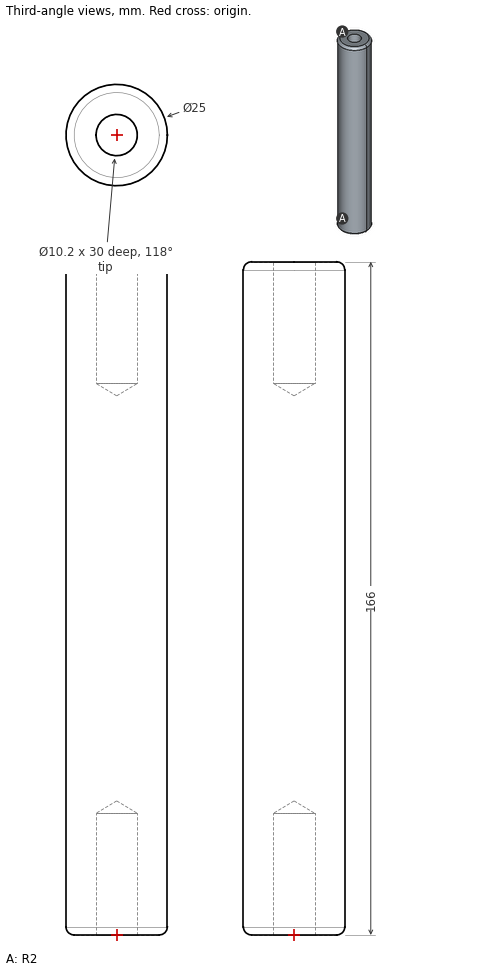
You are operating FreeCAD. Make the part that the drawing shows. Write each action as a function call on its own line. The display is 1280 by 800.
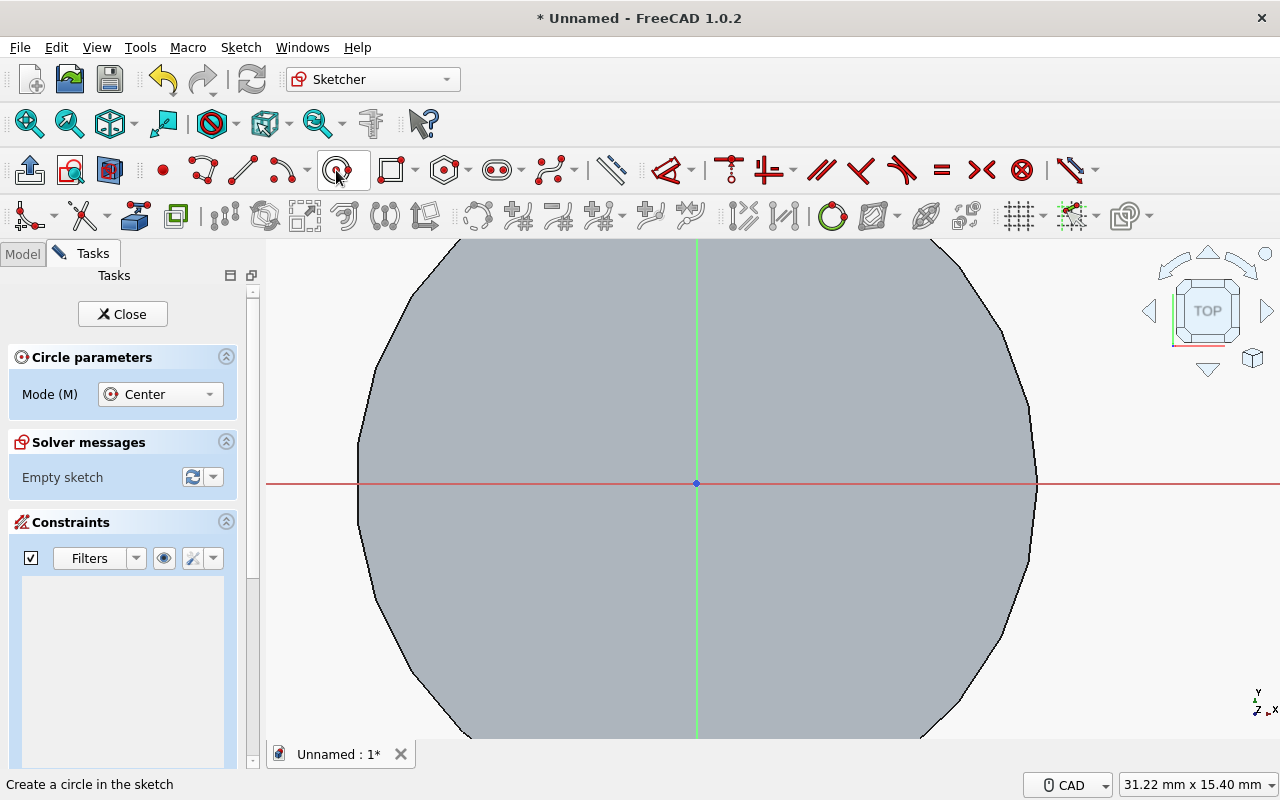
click(697, 484)
click(814, 367)
key(Escape)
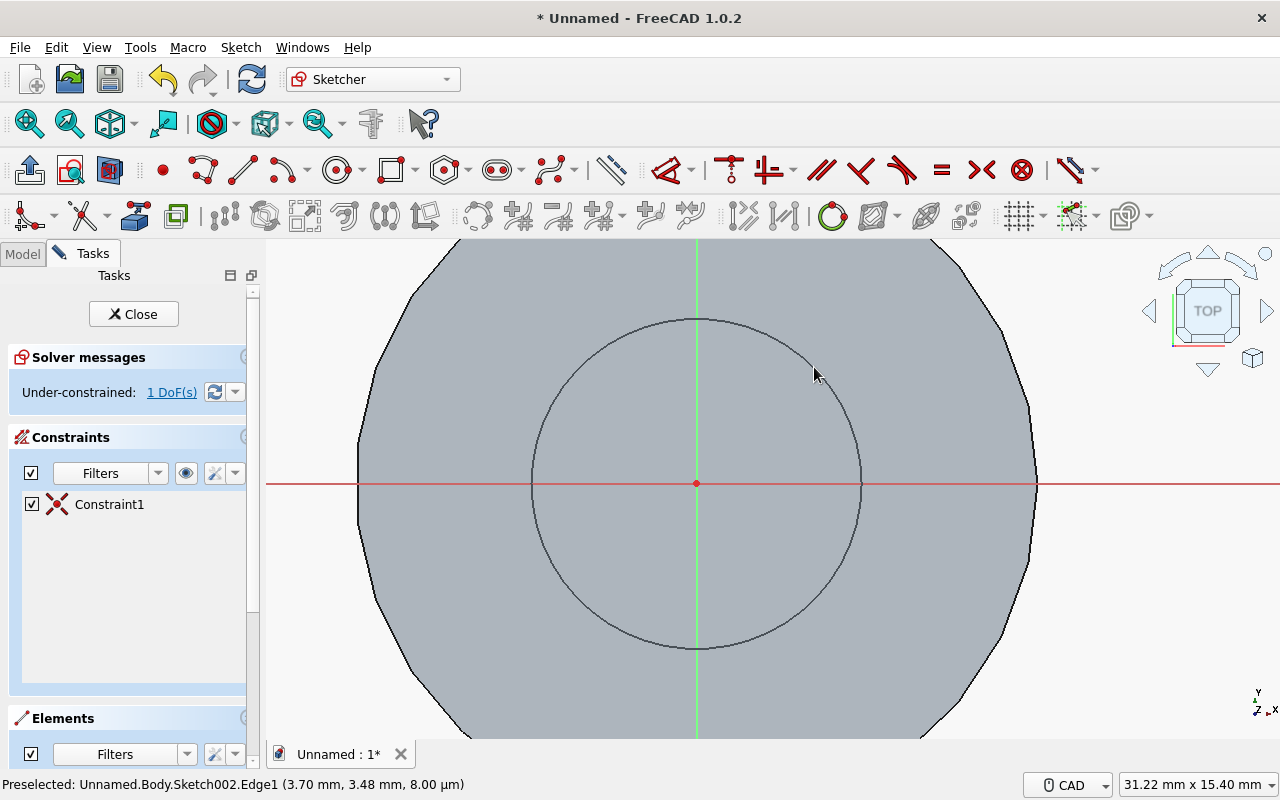
click(666, 170)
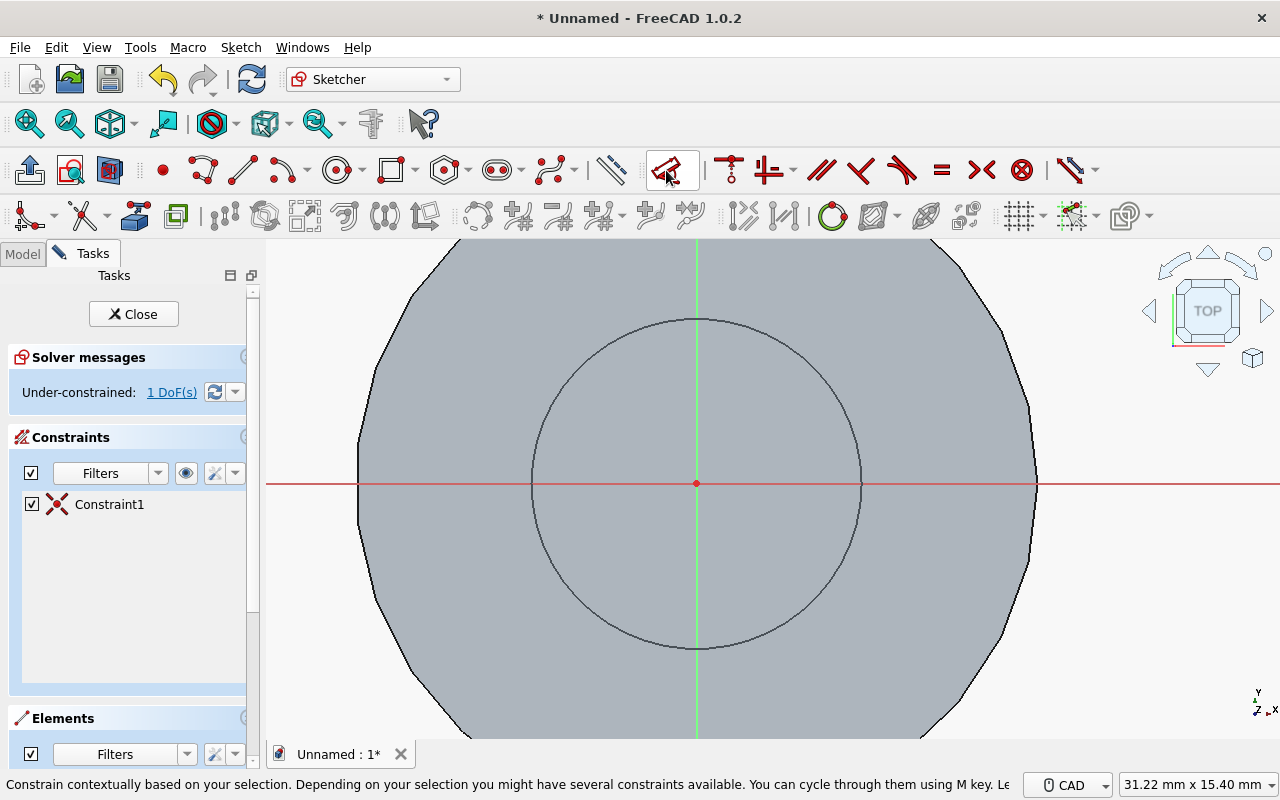
click(813, 367)
click(836, 344)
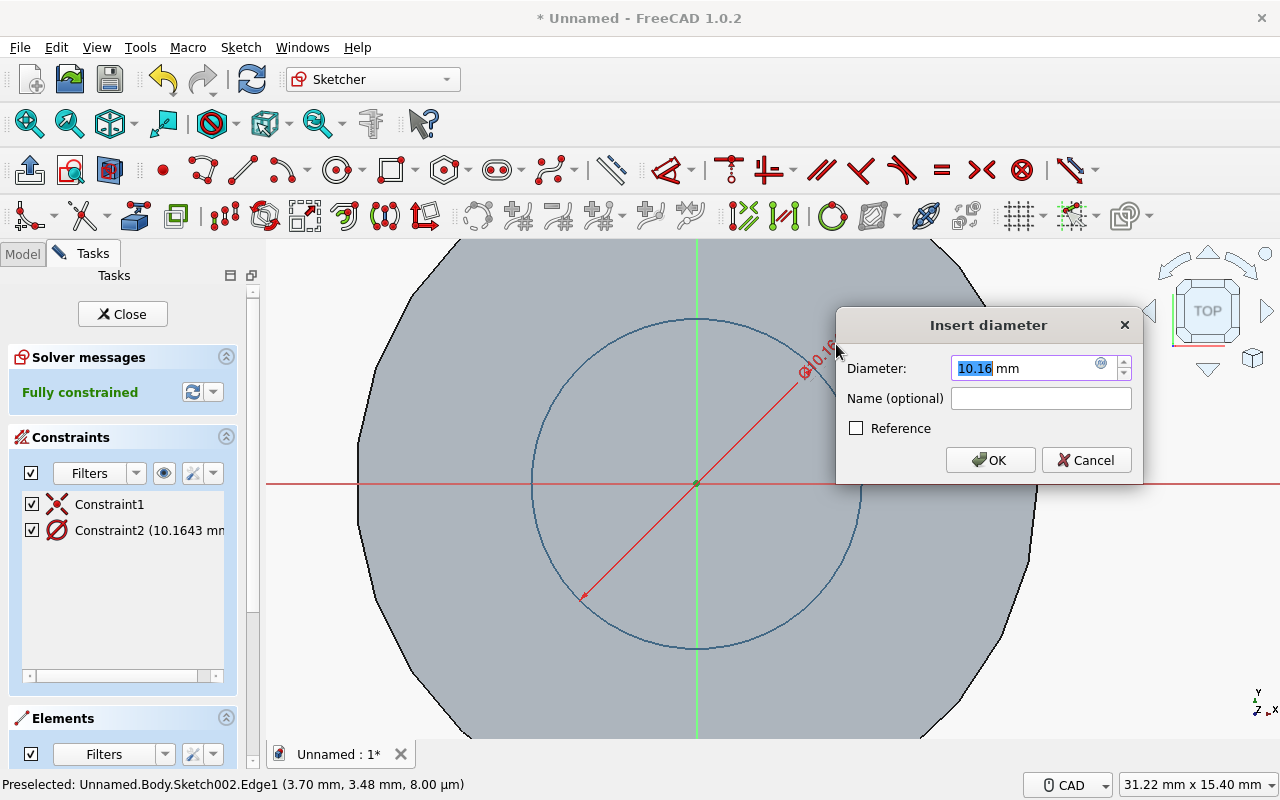
text(10.2)
key(Return)
key(Escape)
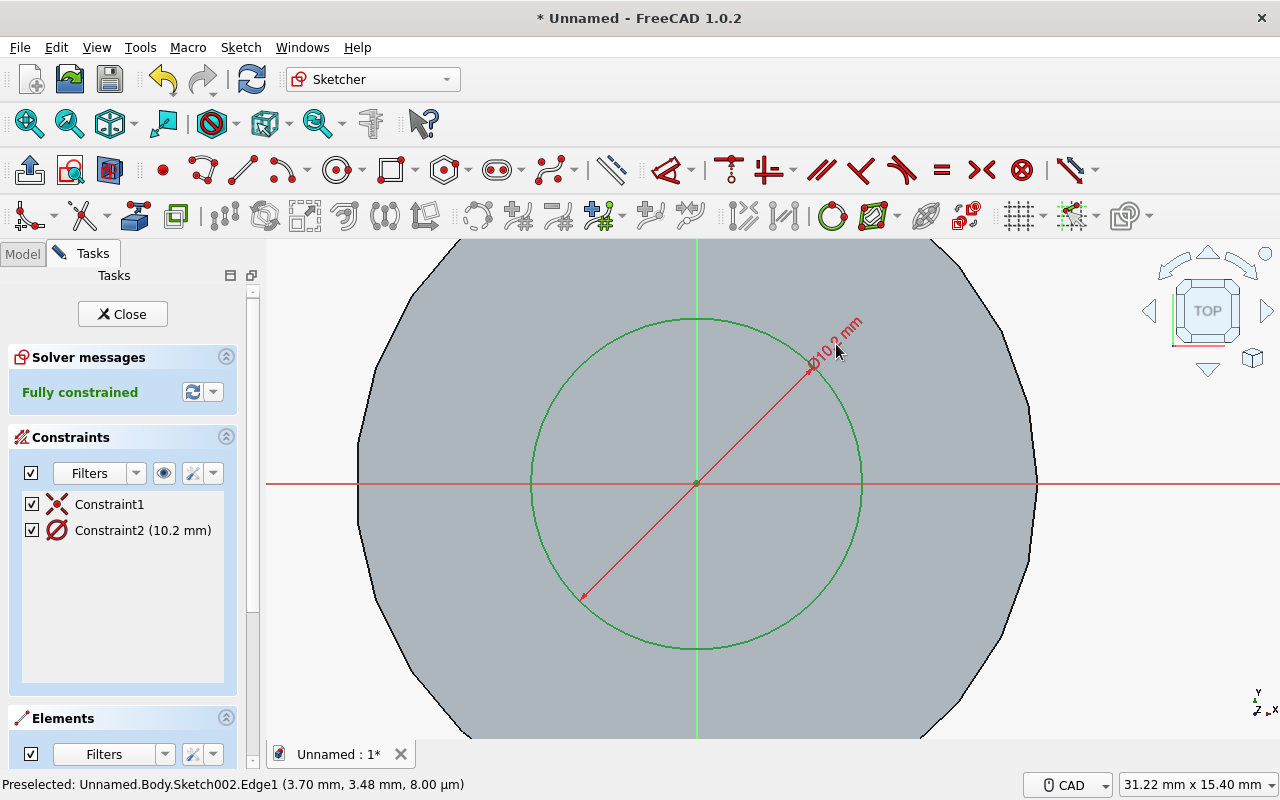
click(123, 314)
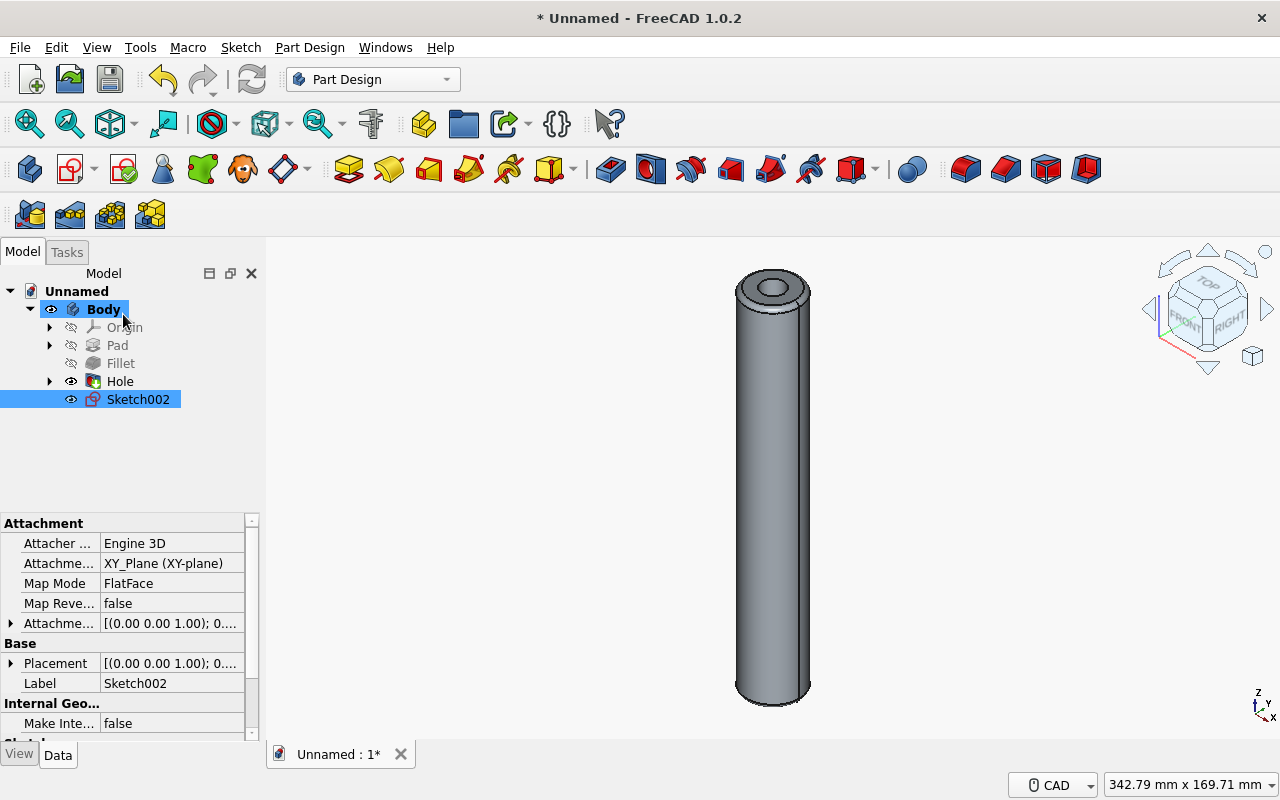
click(652, 170)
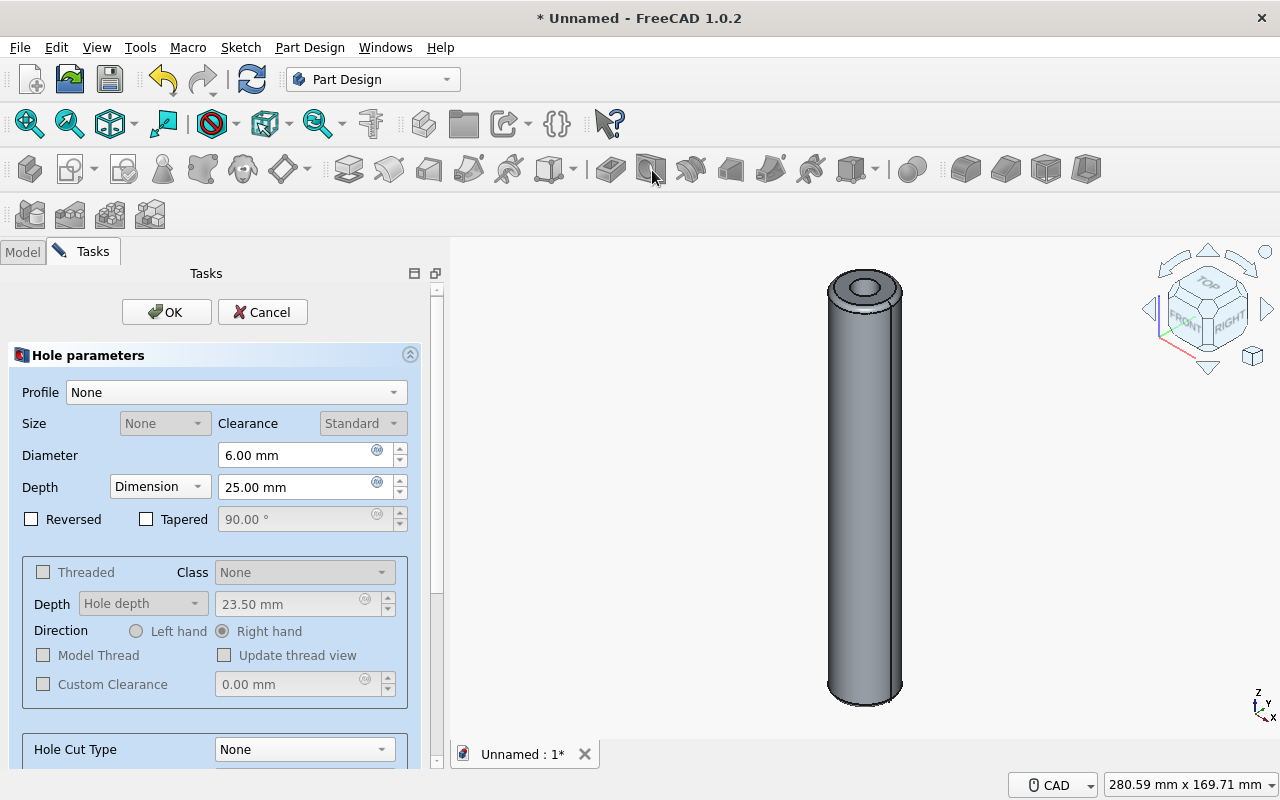
triple_click(305, 455)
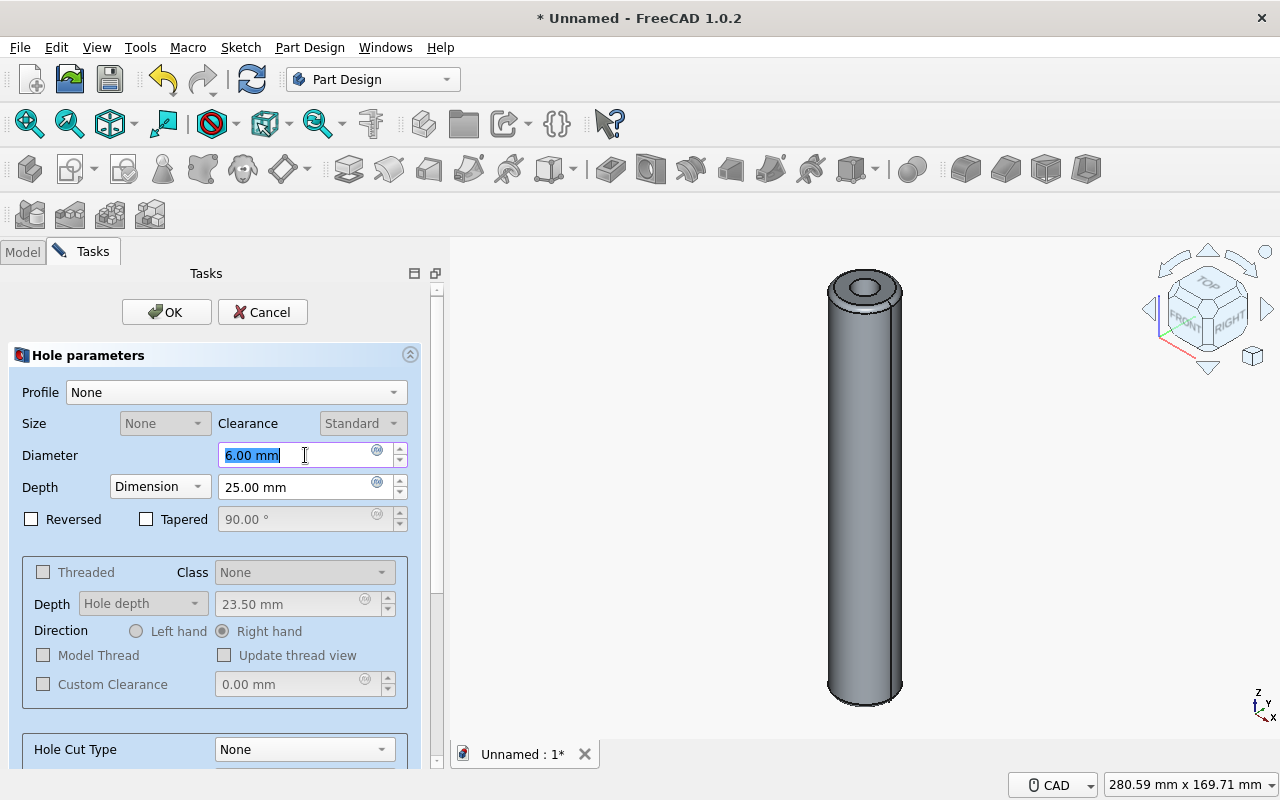
text(10.2)
key(Tab)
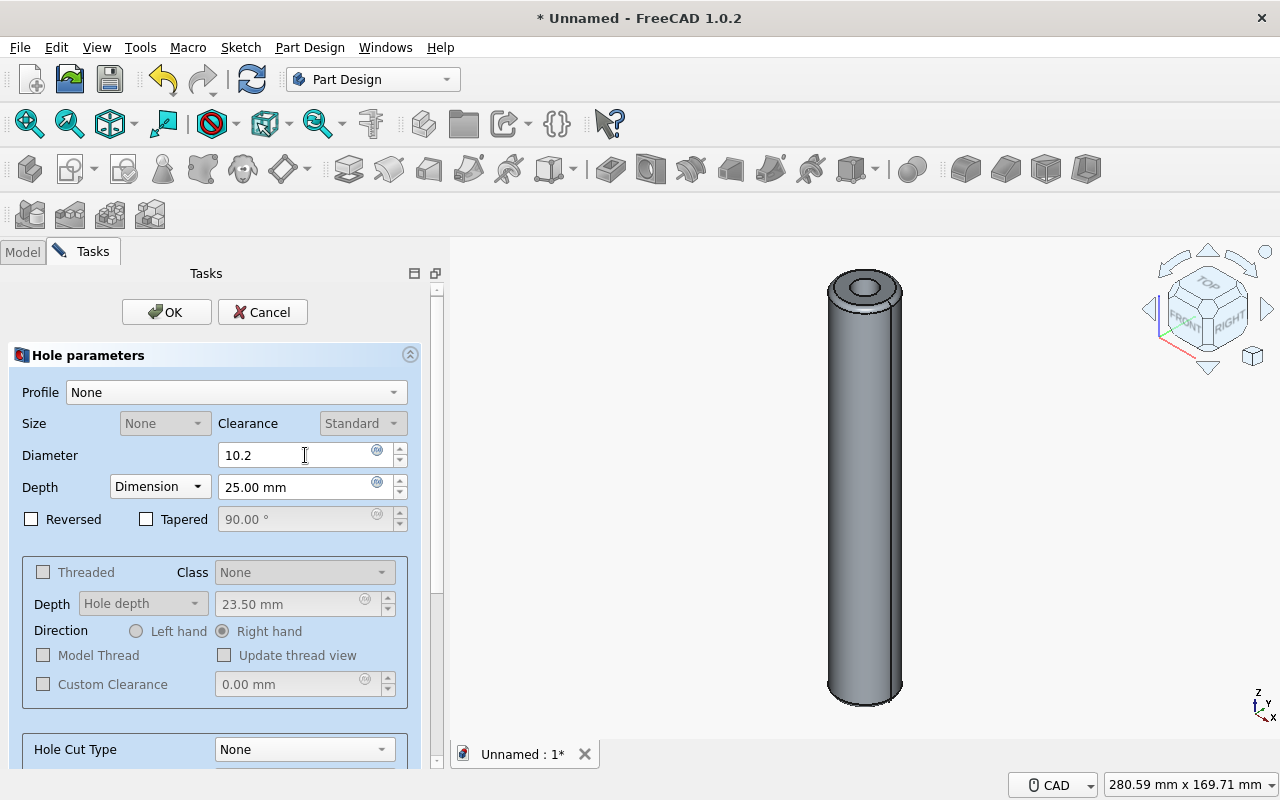
triple_click(305, 487)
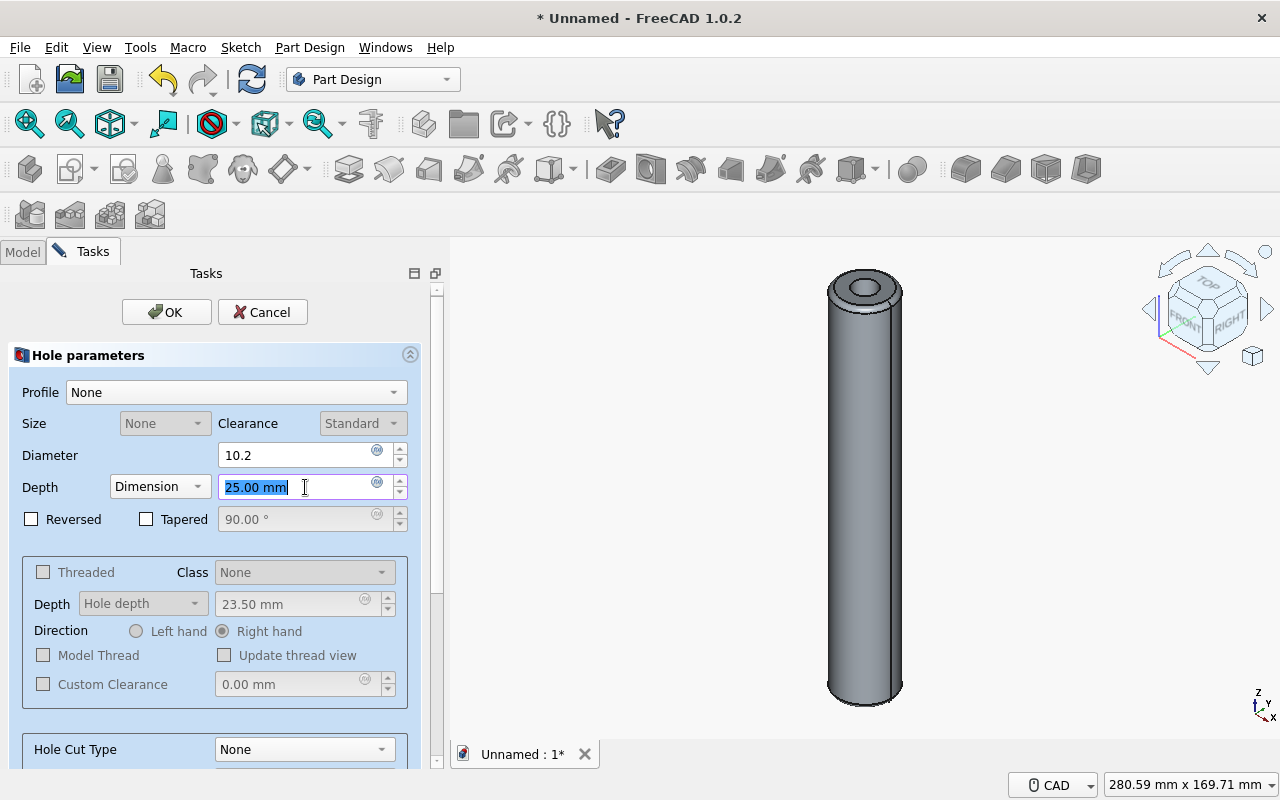
text(30)
key(Tab)